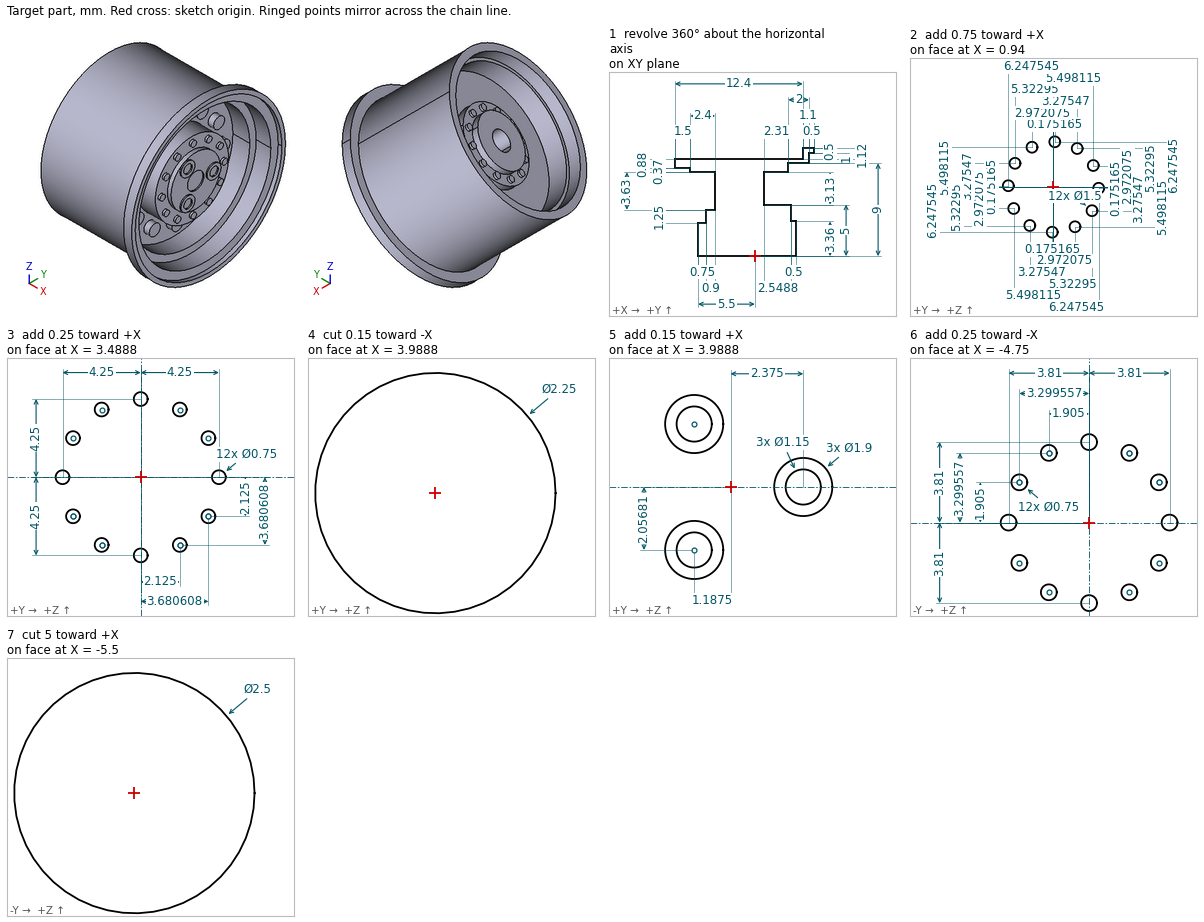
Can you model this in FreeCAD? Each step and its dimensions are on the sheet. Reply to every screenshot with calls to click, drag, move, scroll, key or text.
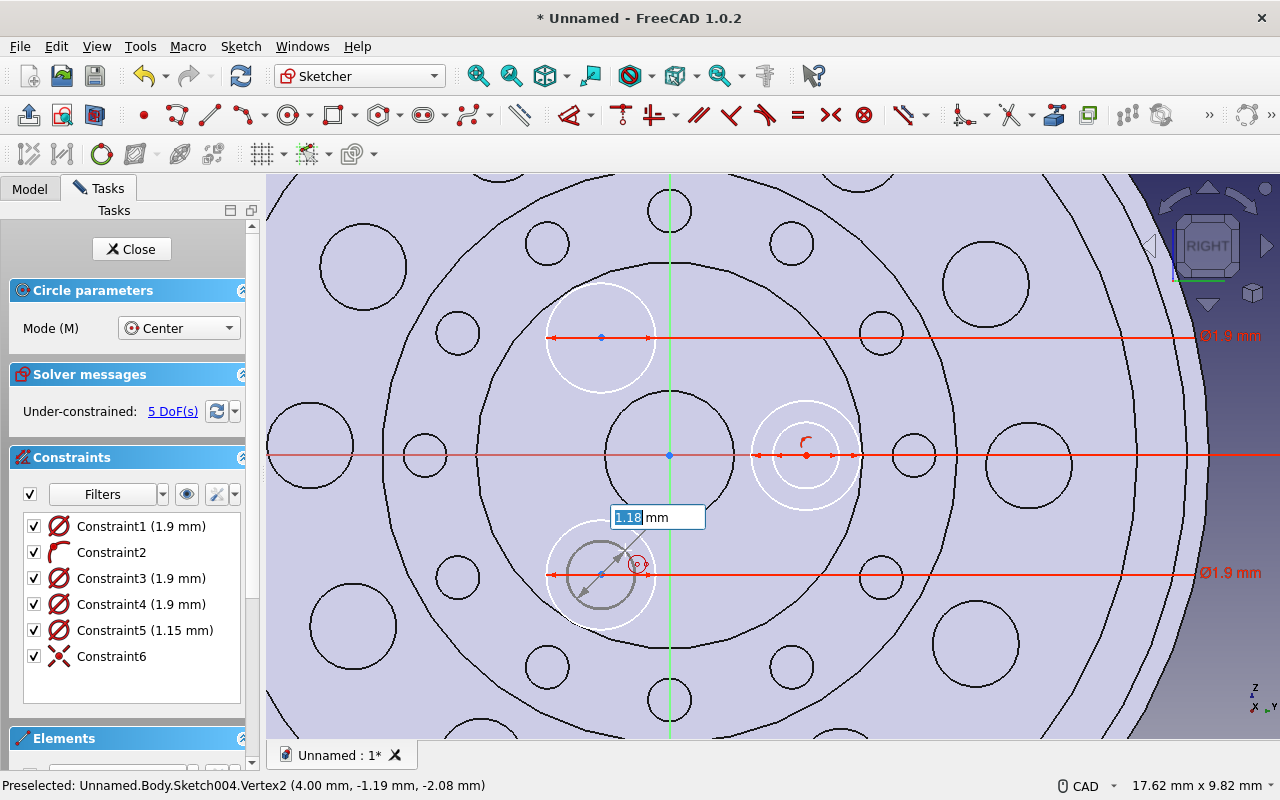
text(1.15)
key(Return)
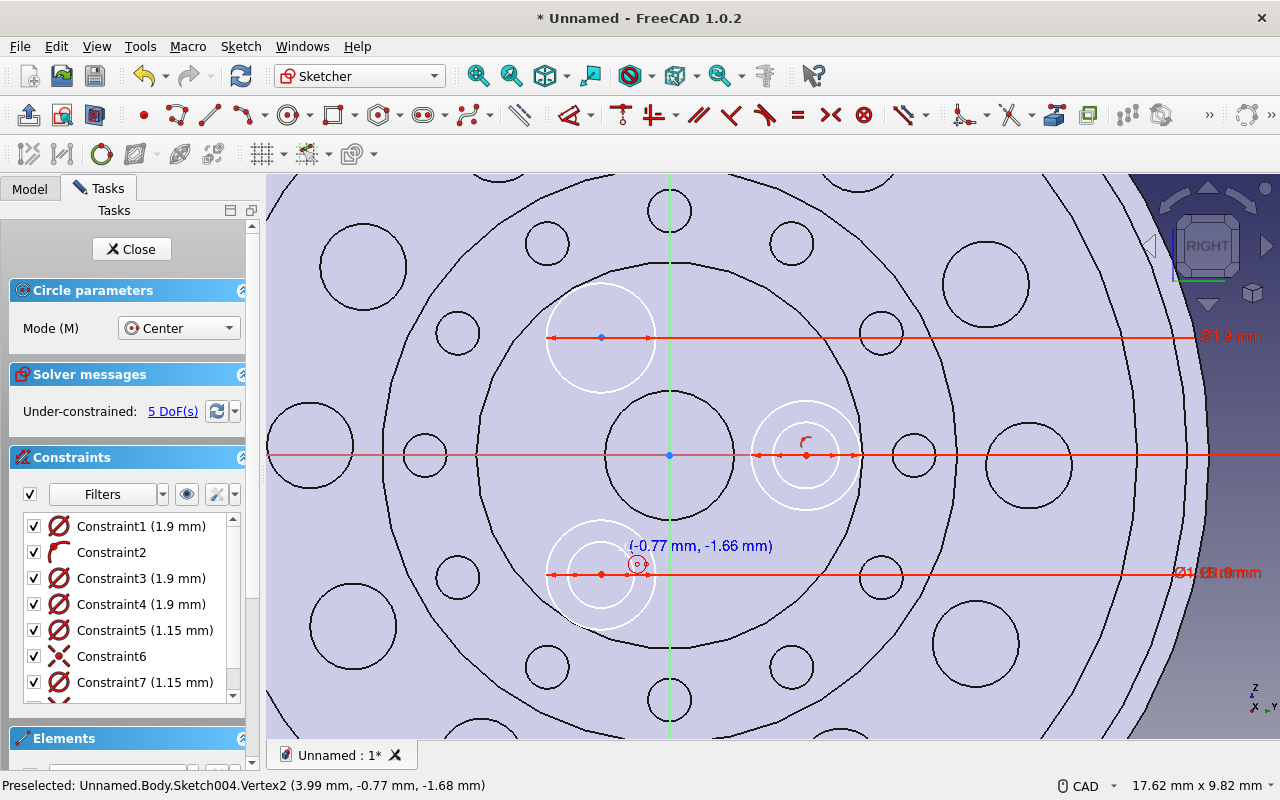
click(601, 338)
move(625, 314)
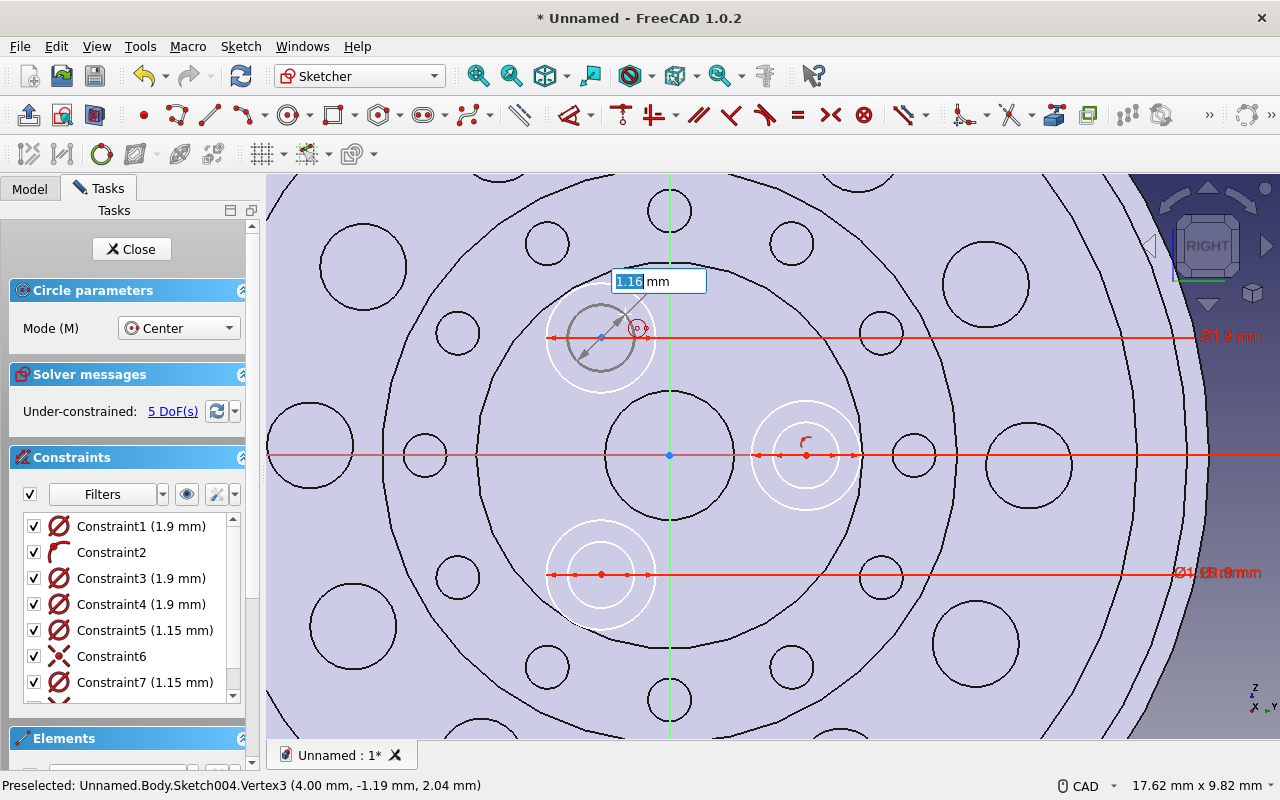
text(1.15)
key(Return)
key(Escape)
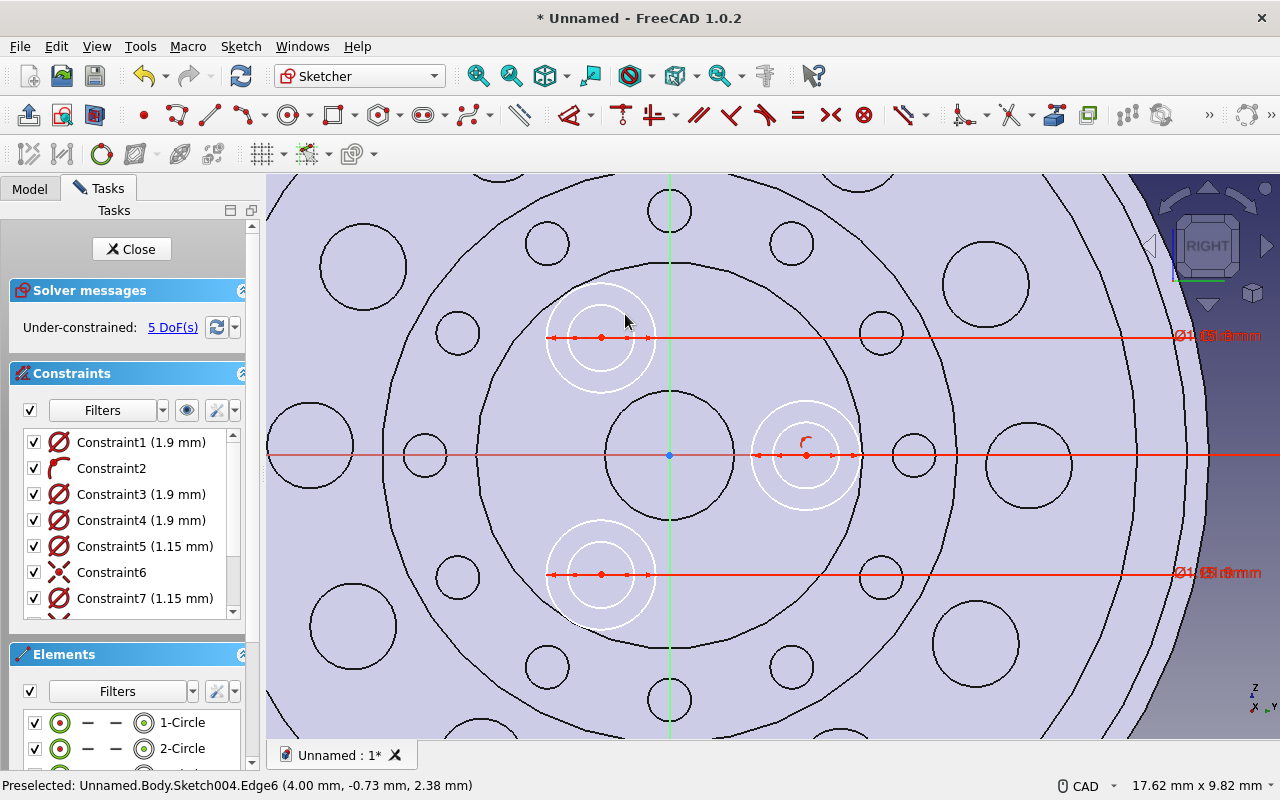
click(601, 575)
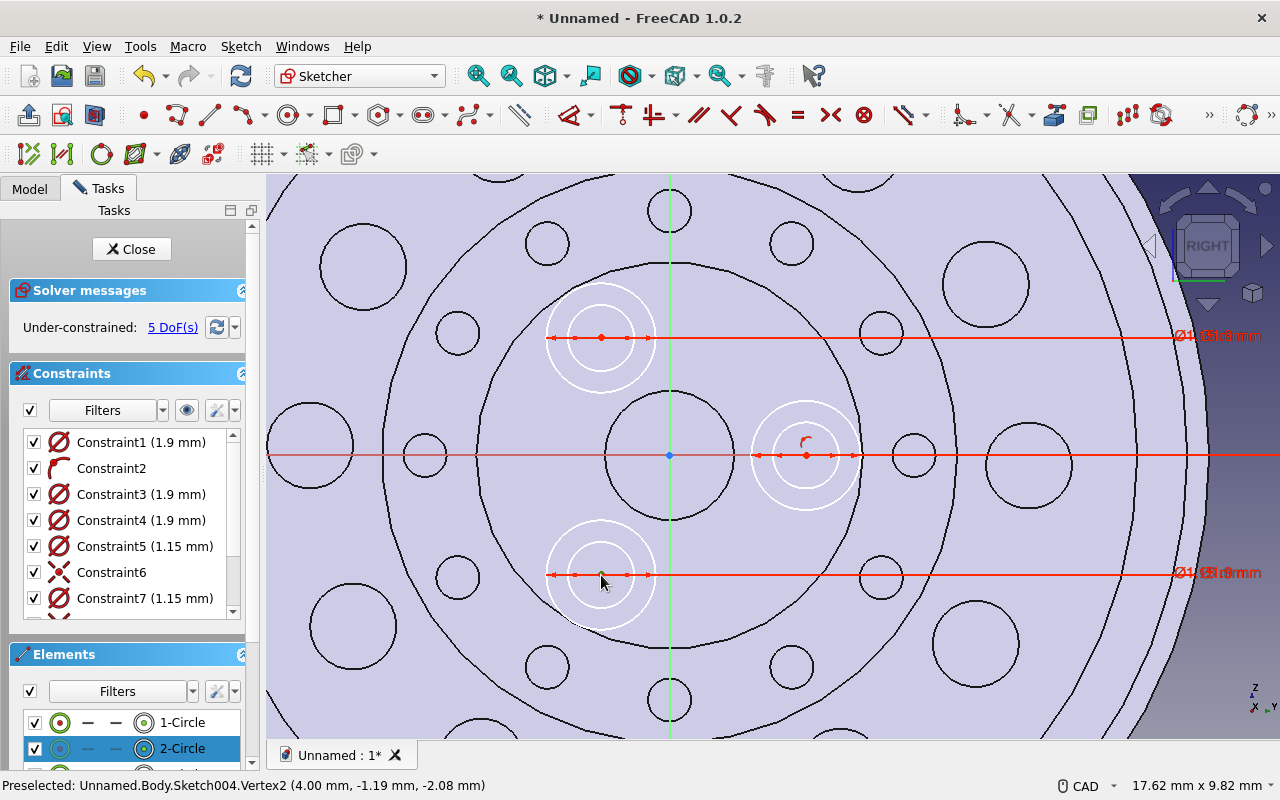
click(601, 338)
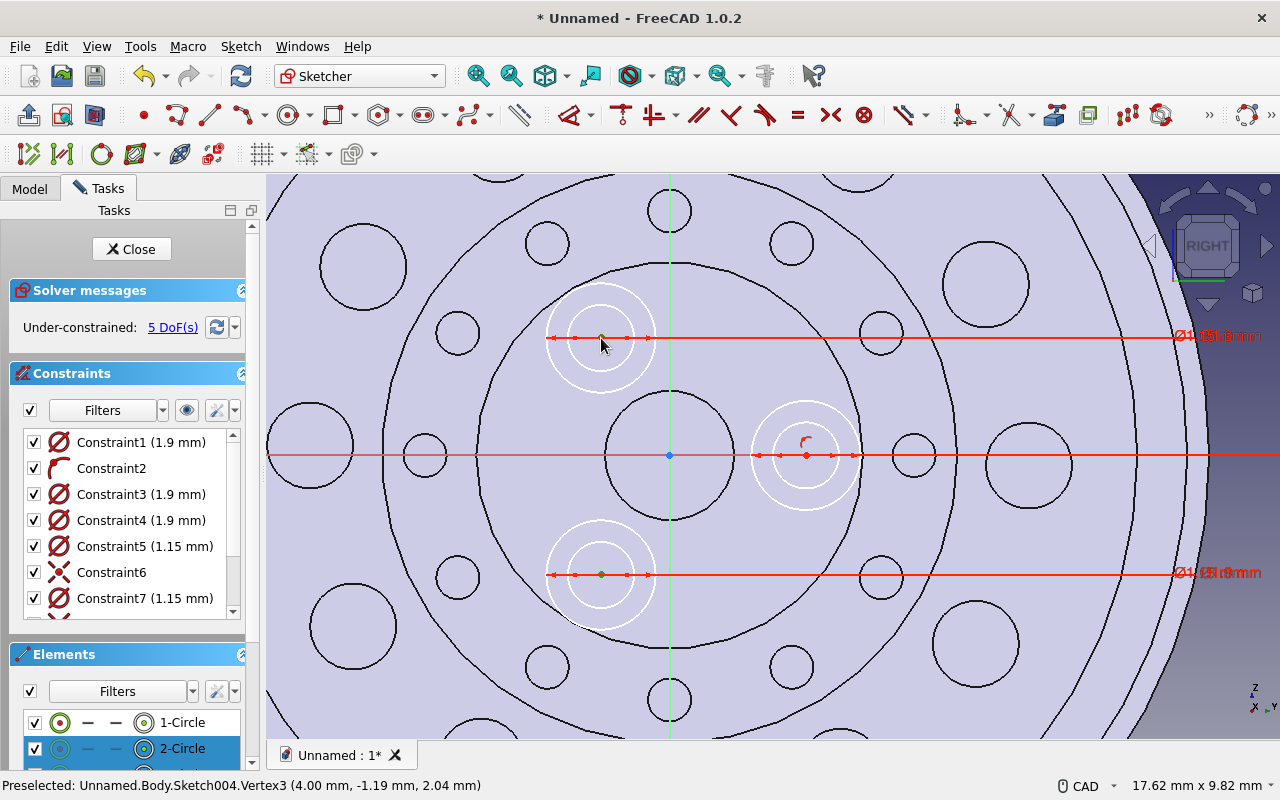
click(353, 455)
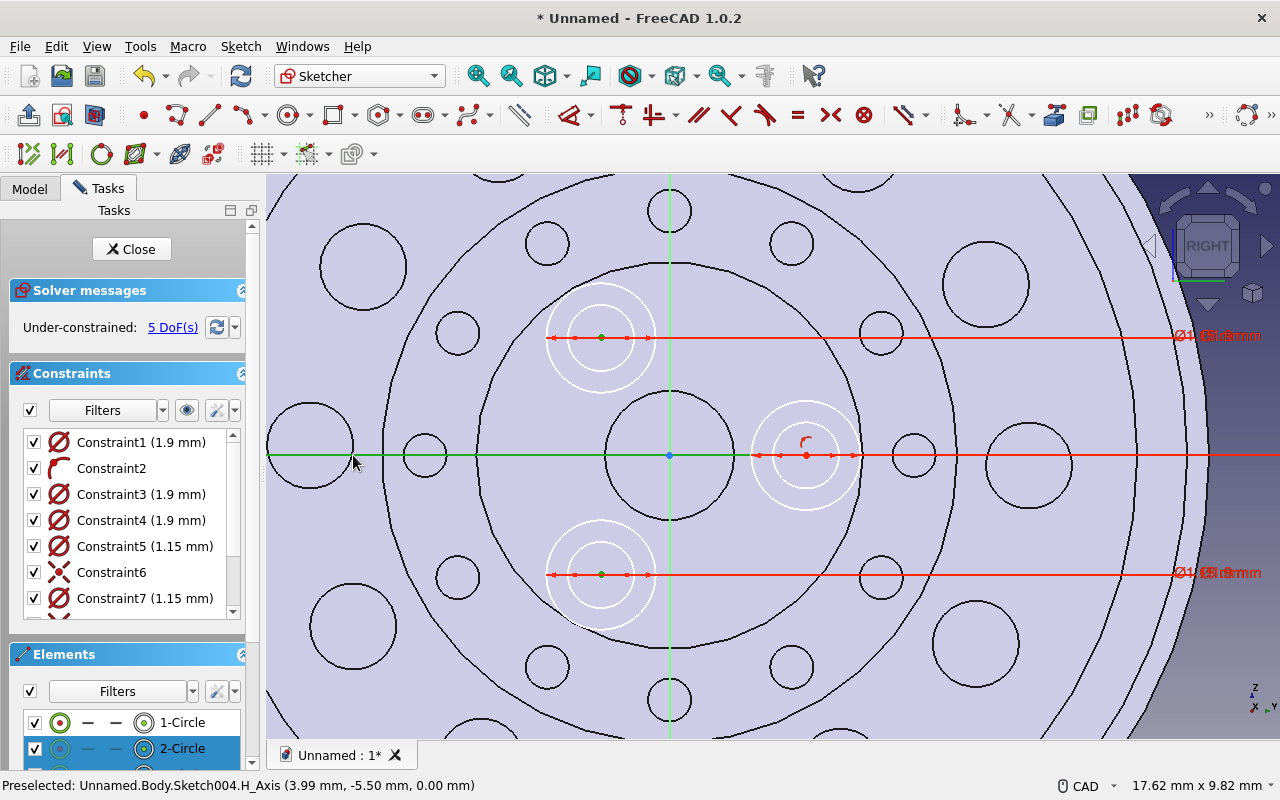
click(831, 116)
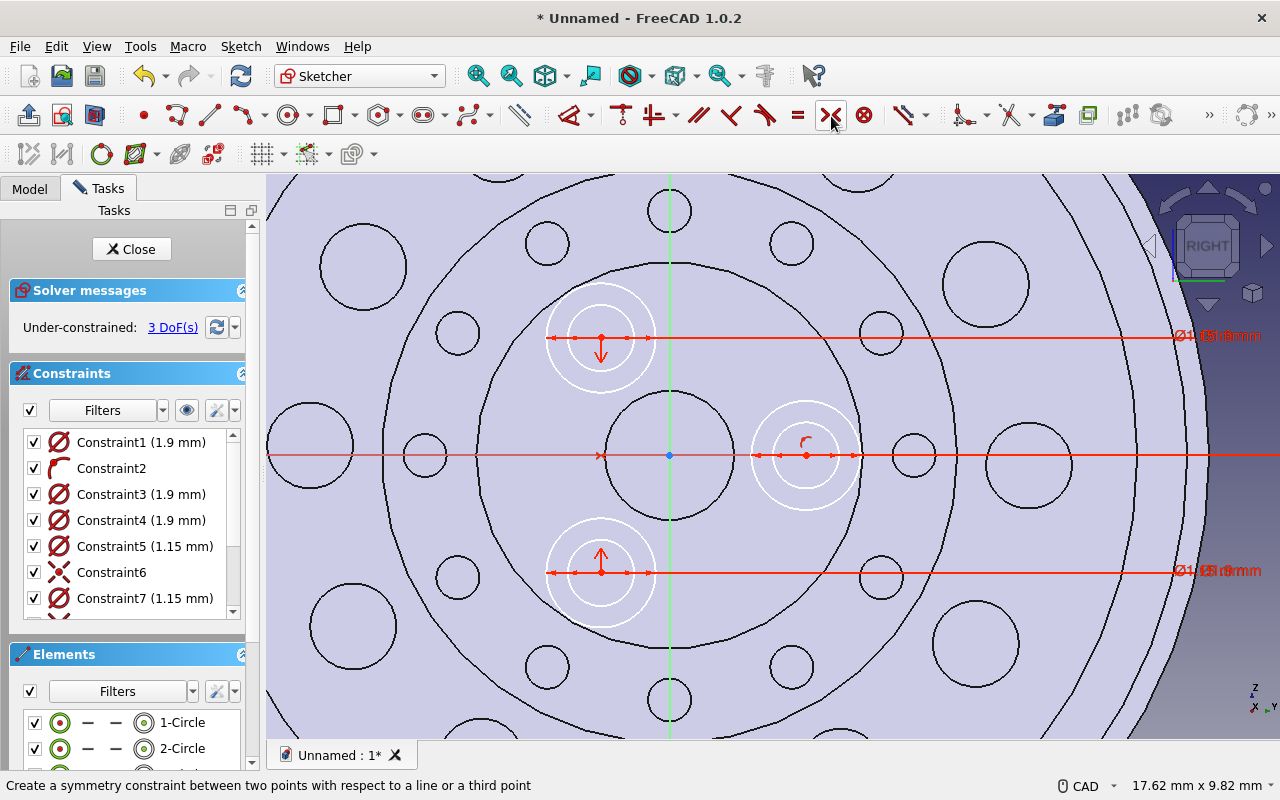
click(568, 116)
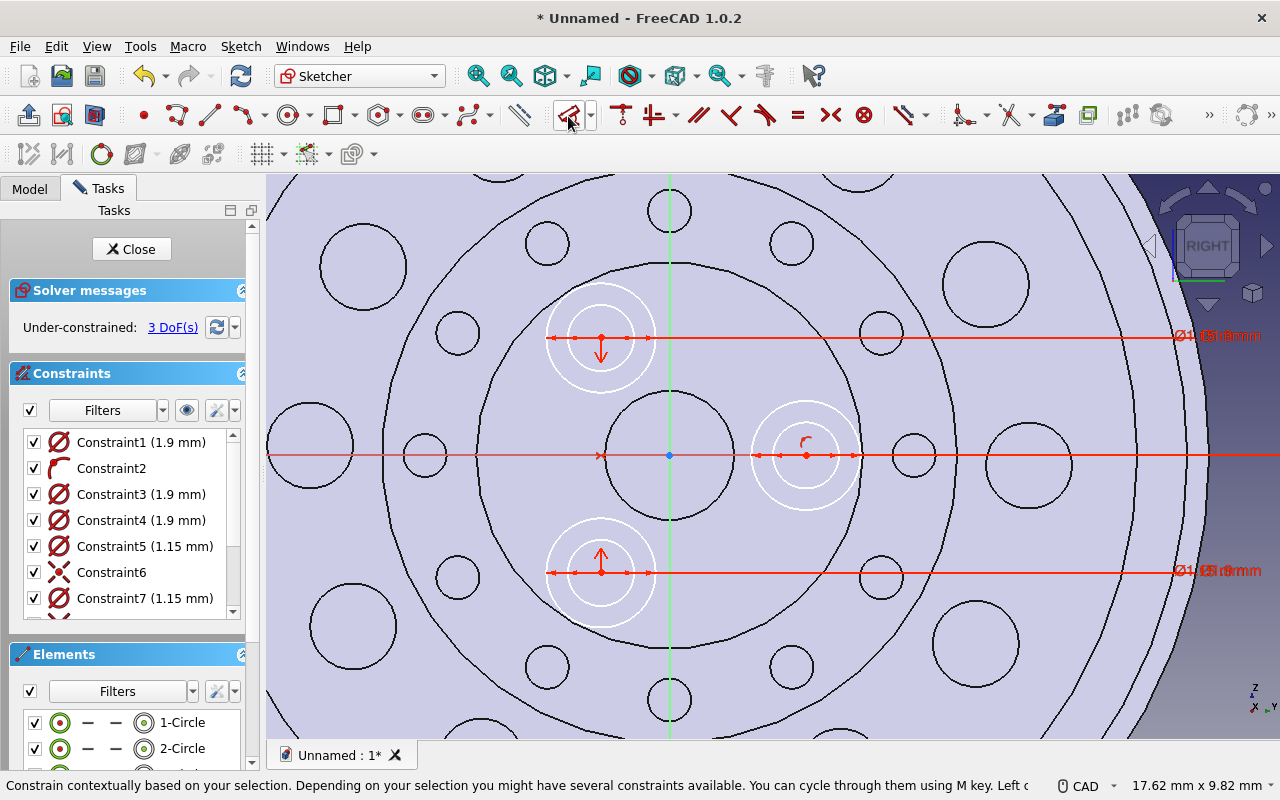
click(806, 455)
click(738, 489)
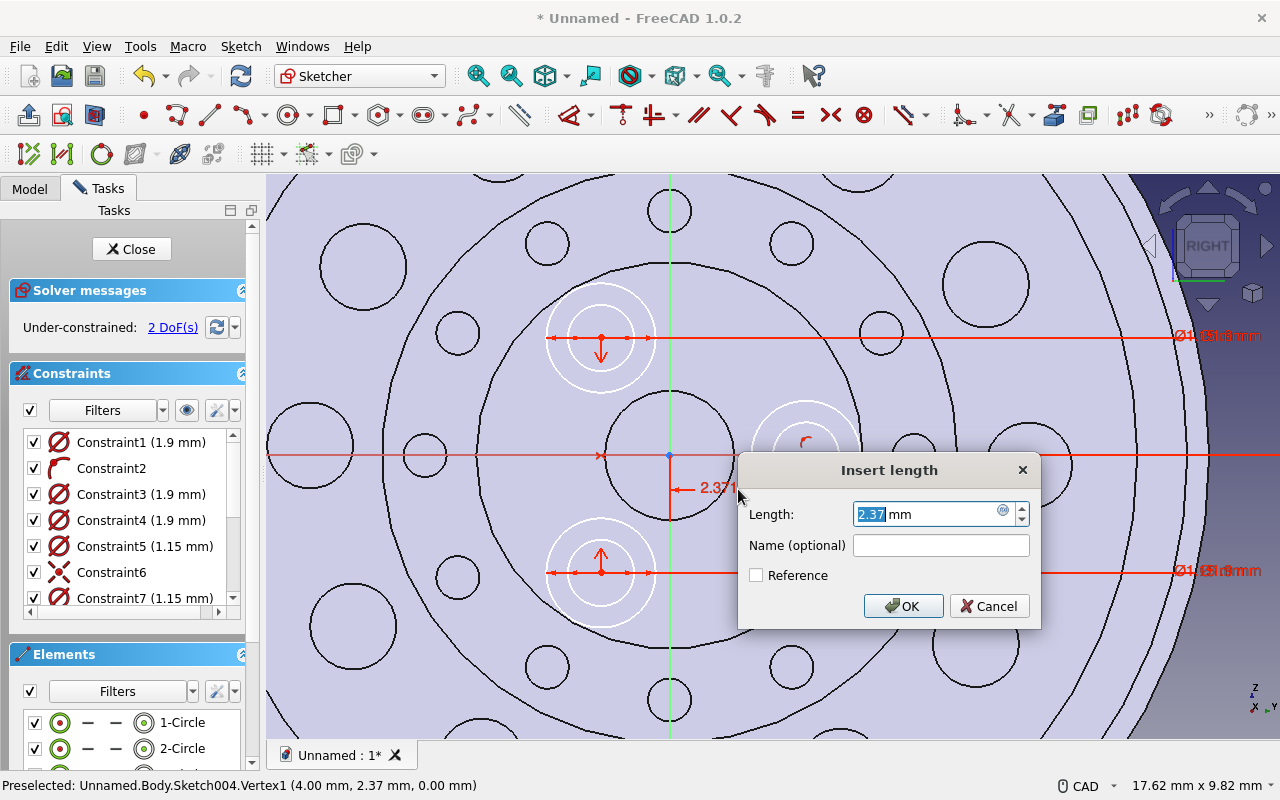
text(2.375)
key(Return)